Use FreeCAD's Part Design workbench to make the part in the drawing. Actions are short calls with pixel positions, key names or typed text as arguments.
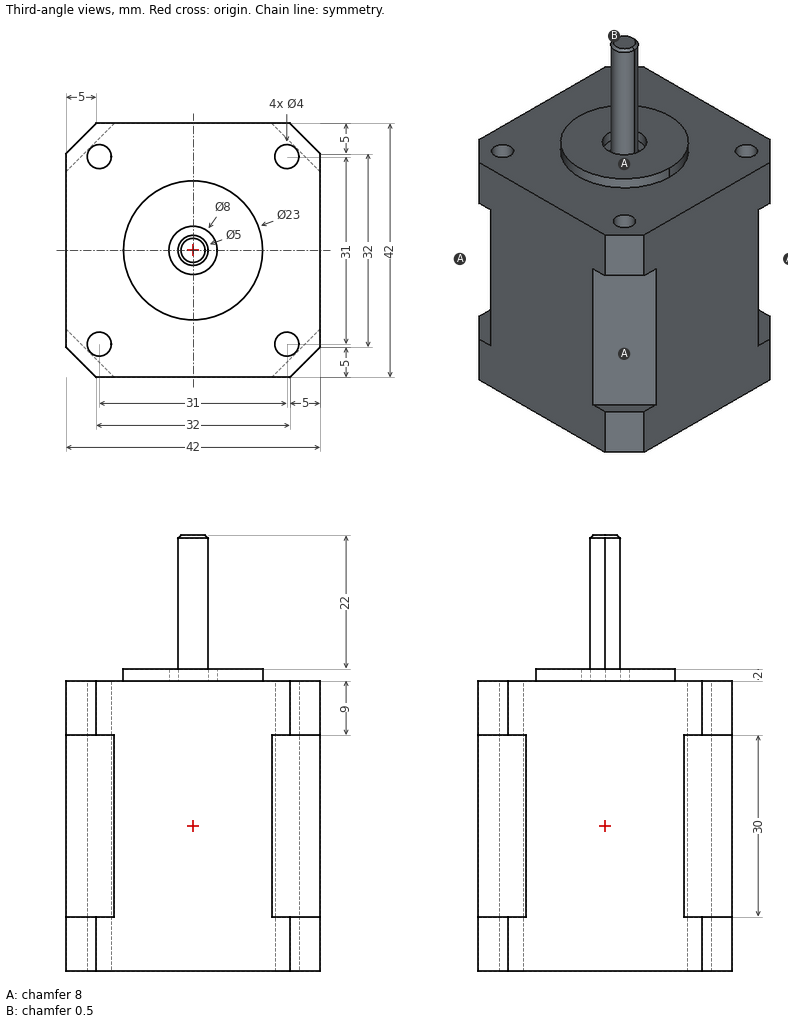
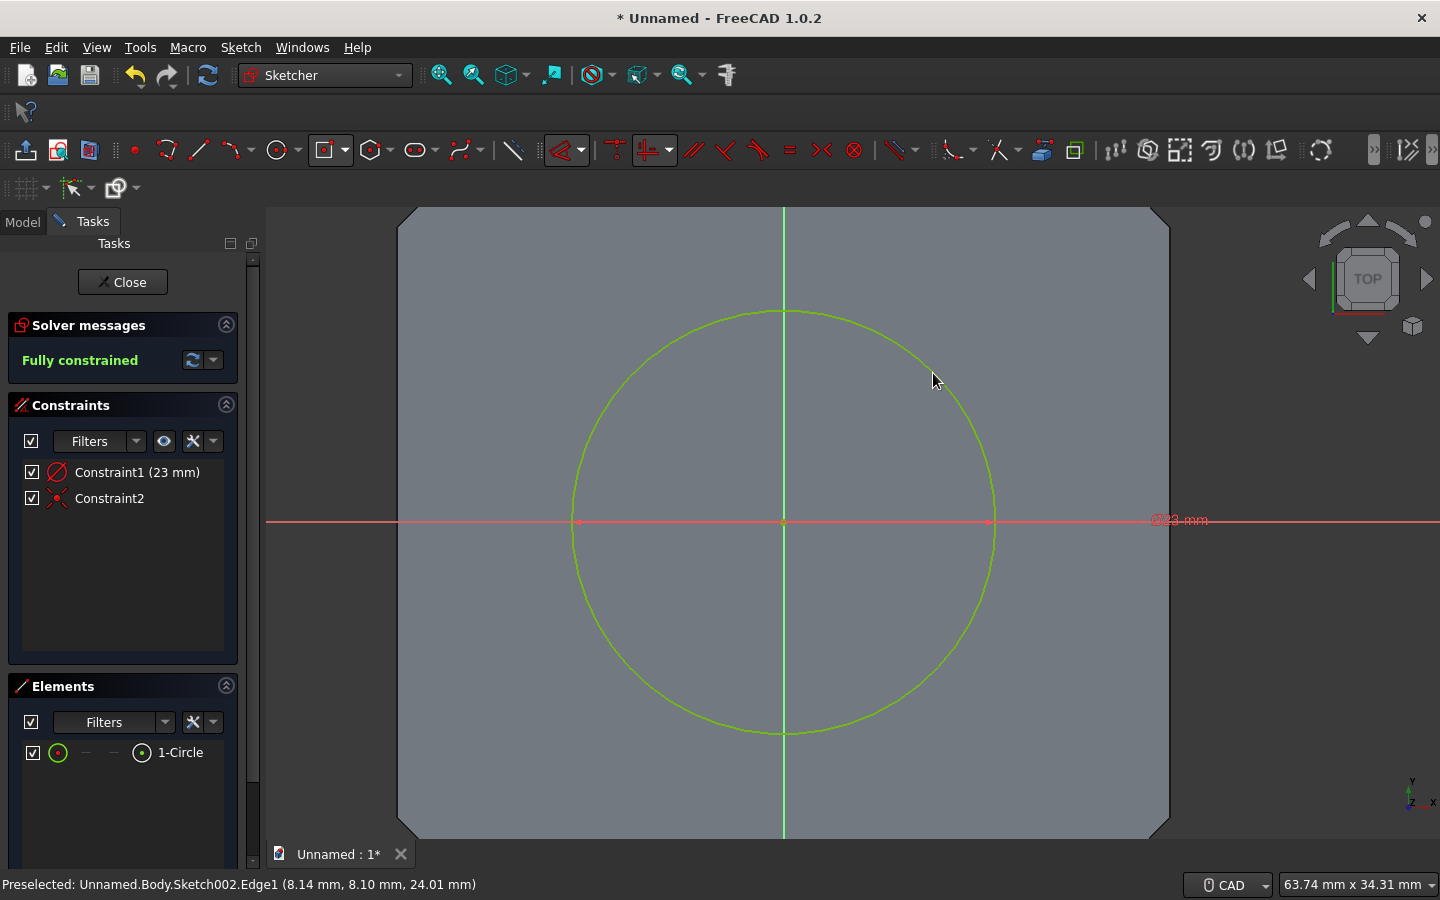
click(123, 282)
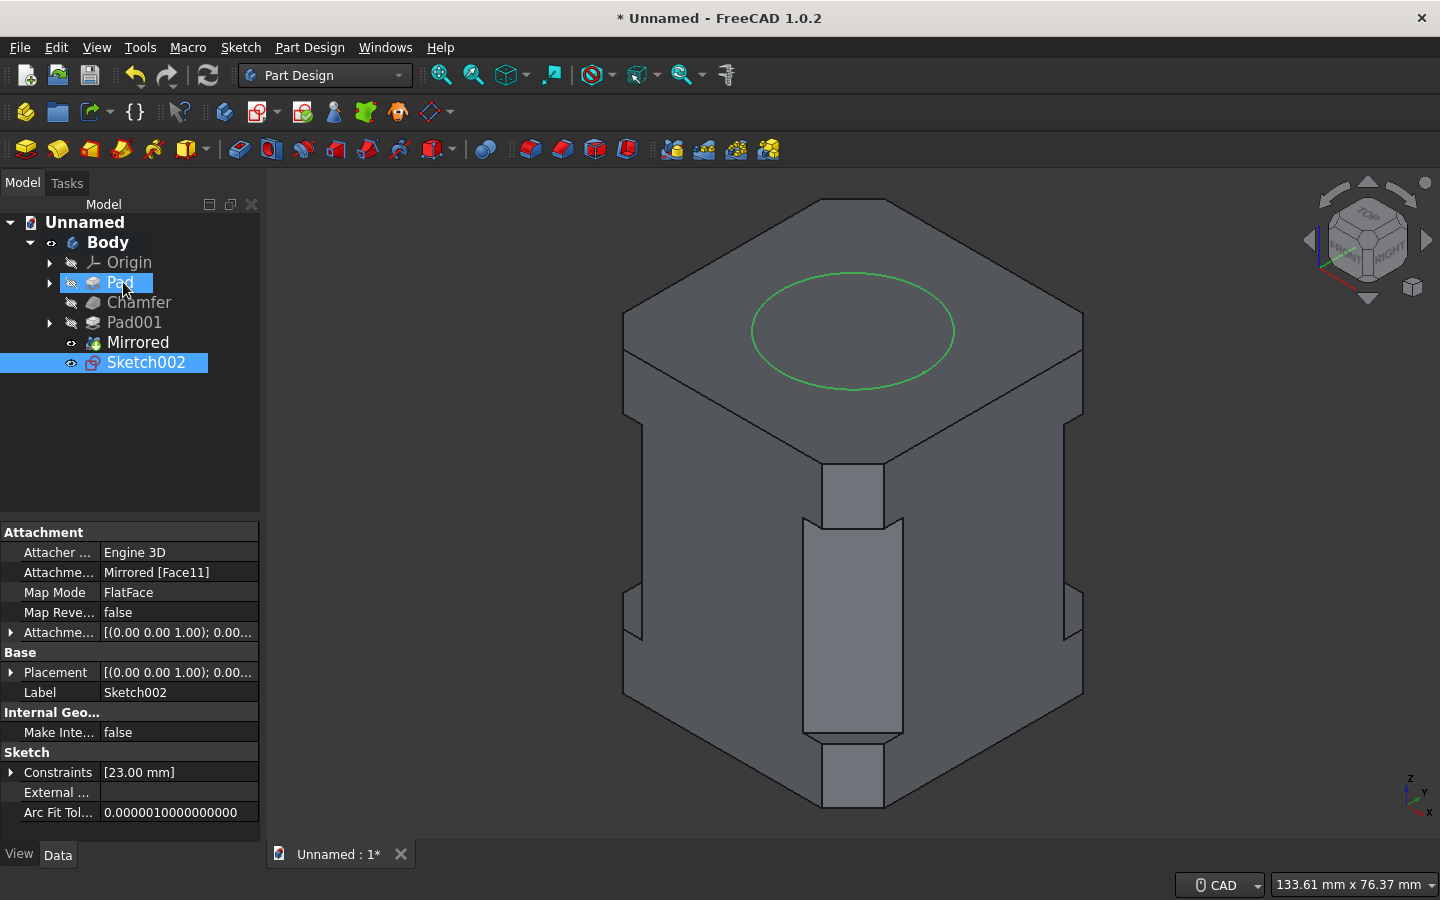
click(26, 150)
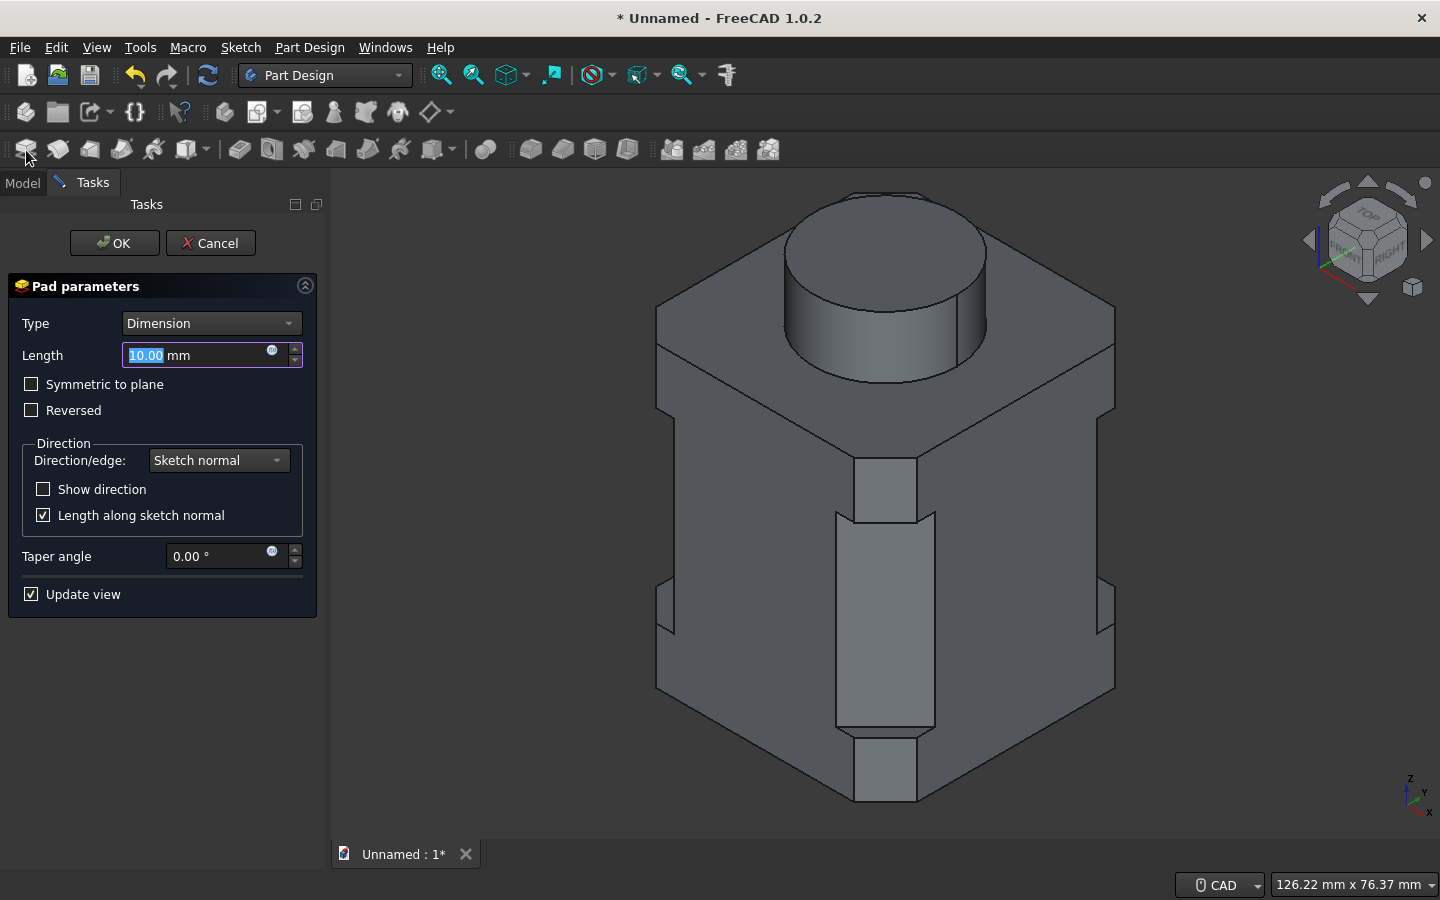
text(2)
key(Tab)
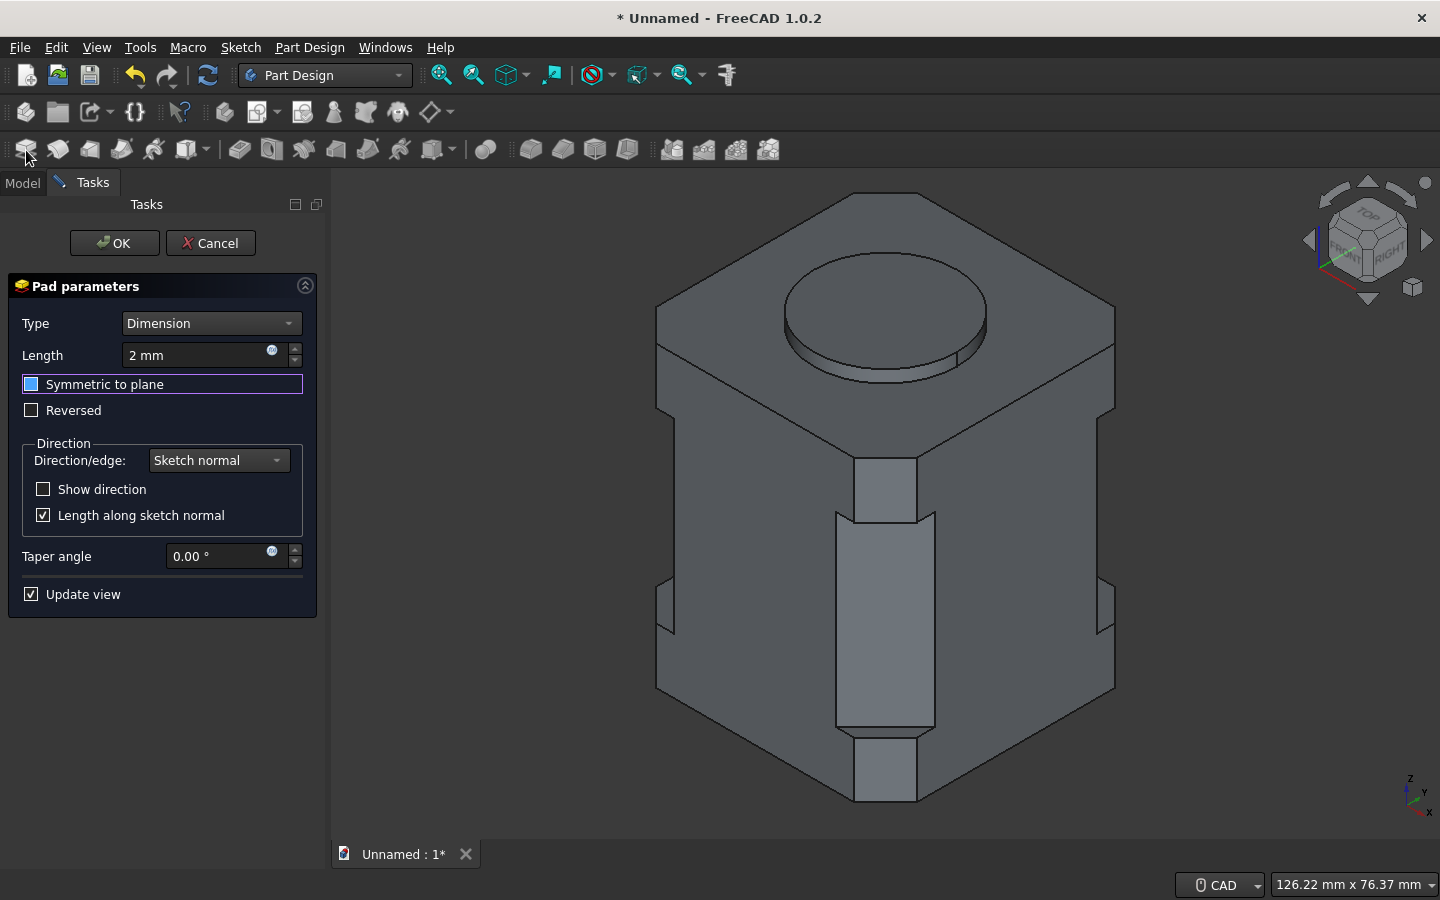
click(115, 243)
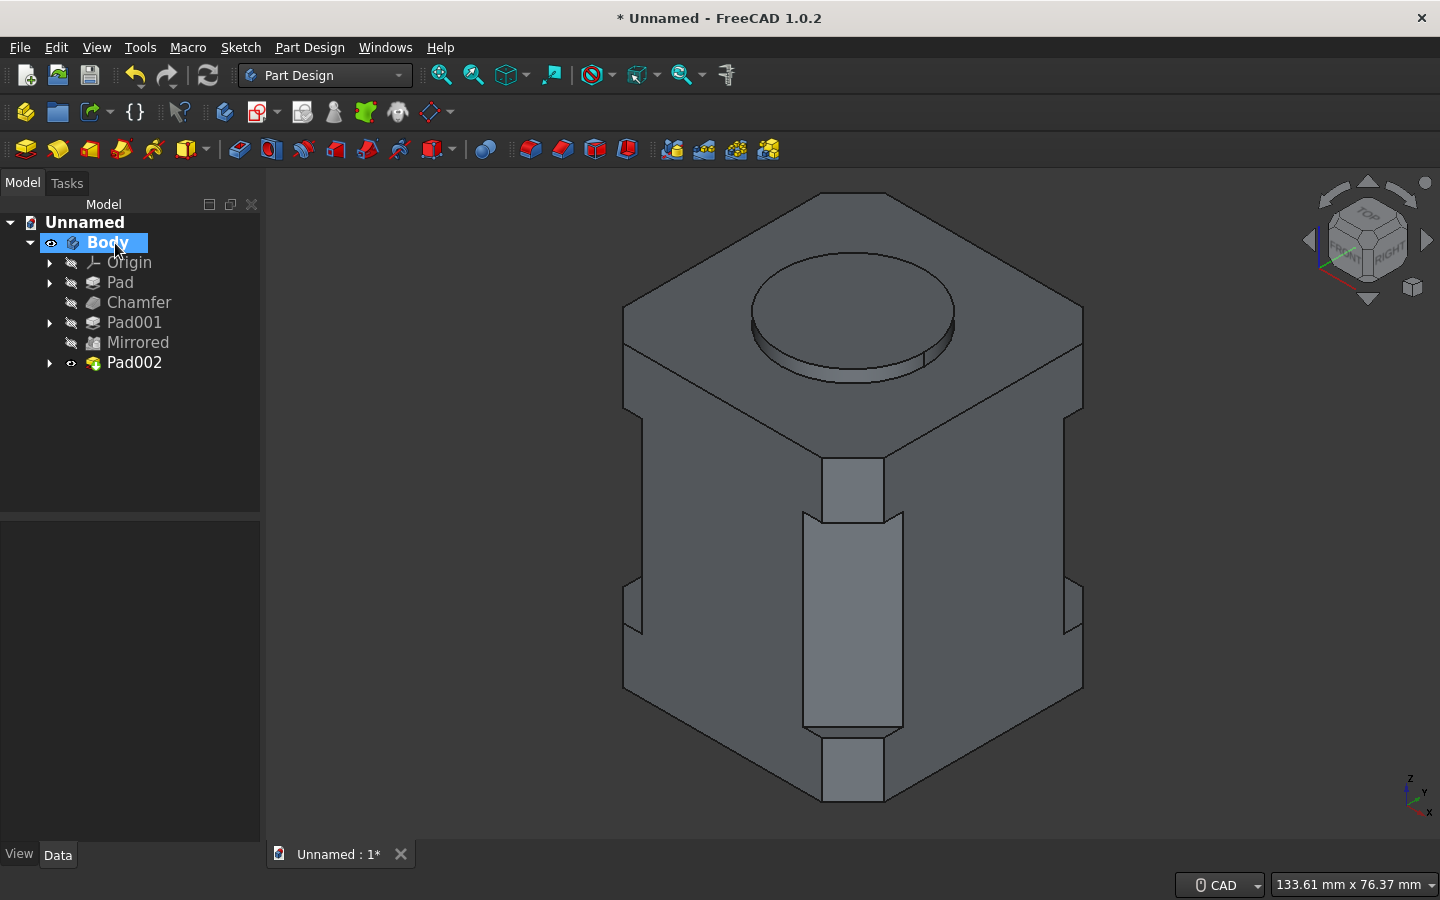
click(442, 76)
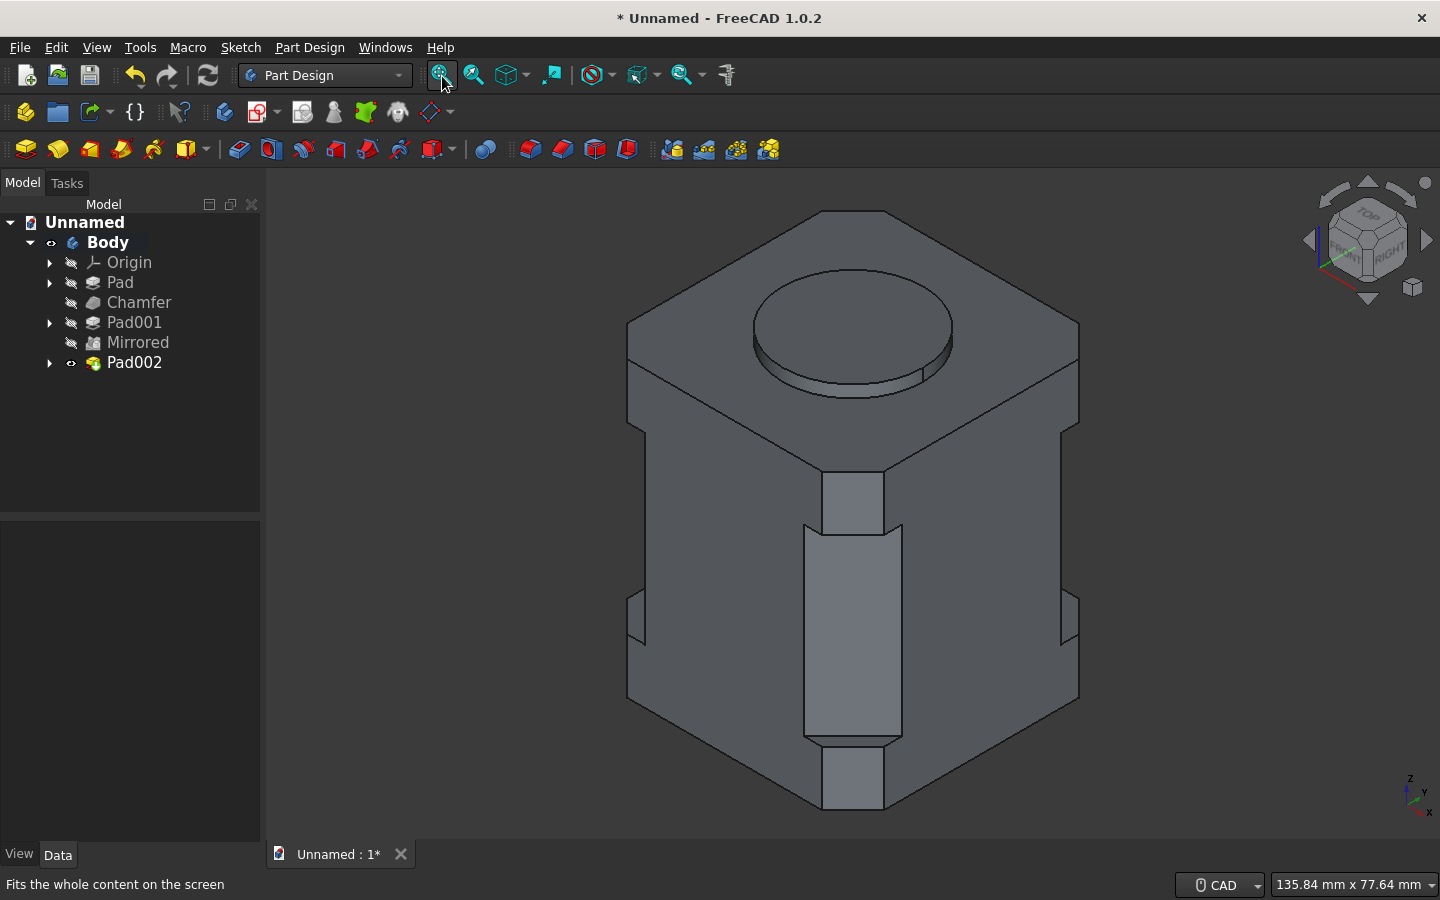
click(853, 326)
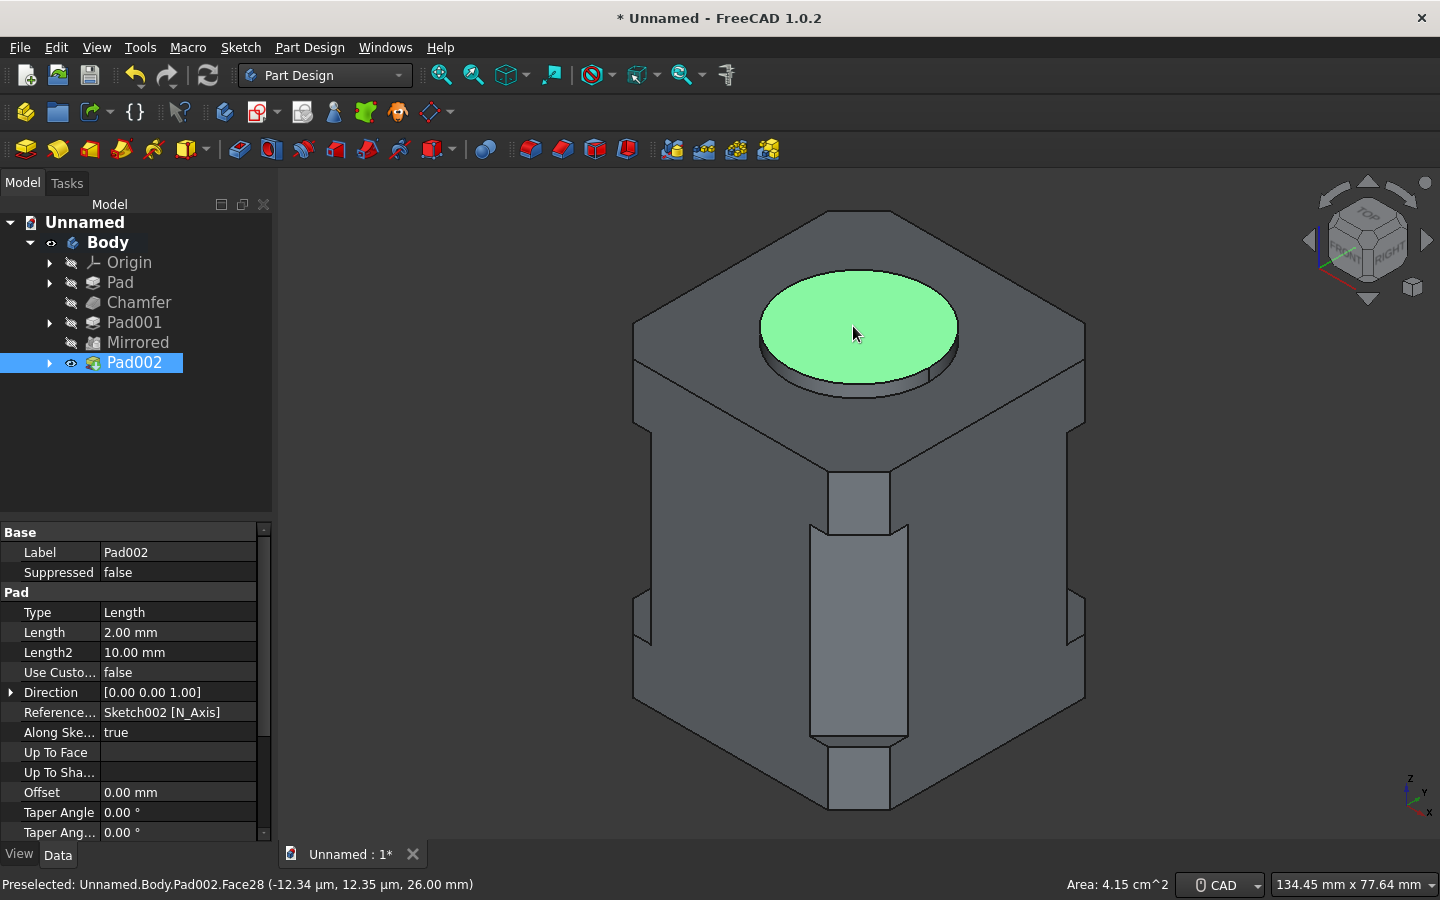
click(258, 112)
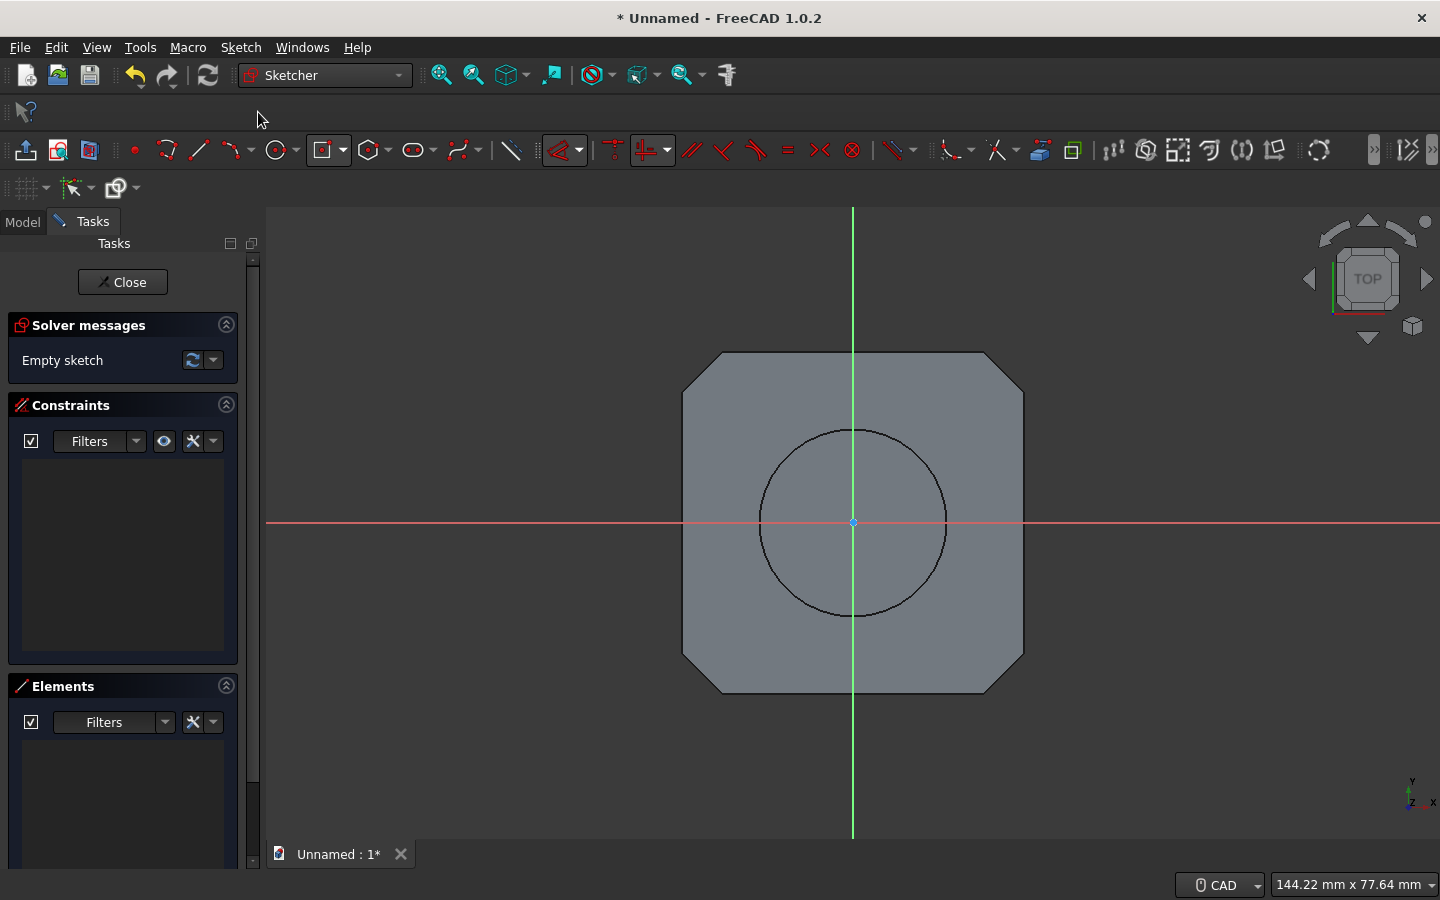
scroll(860, 523, up, 12)